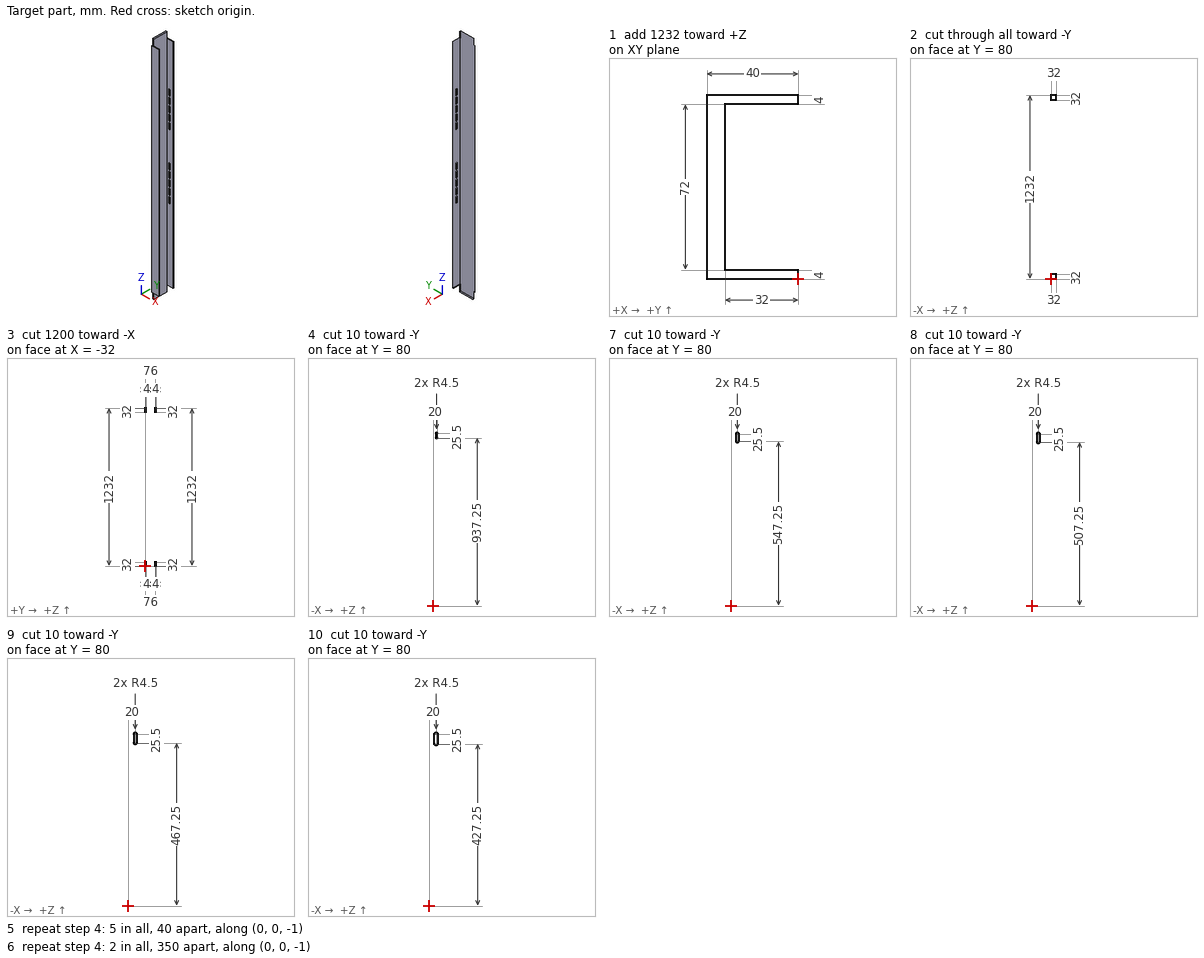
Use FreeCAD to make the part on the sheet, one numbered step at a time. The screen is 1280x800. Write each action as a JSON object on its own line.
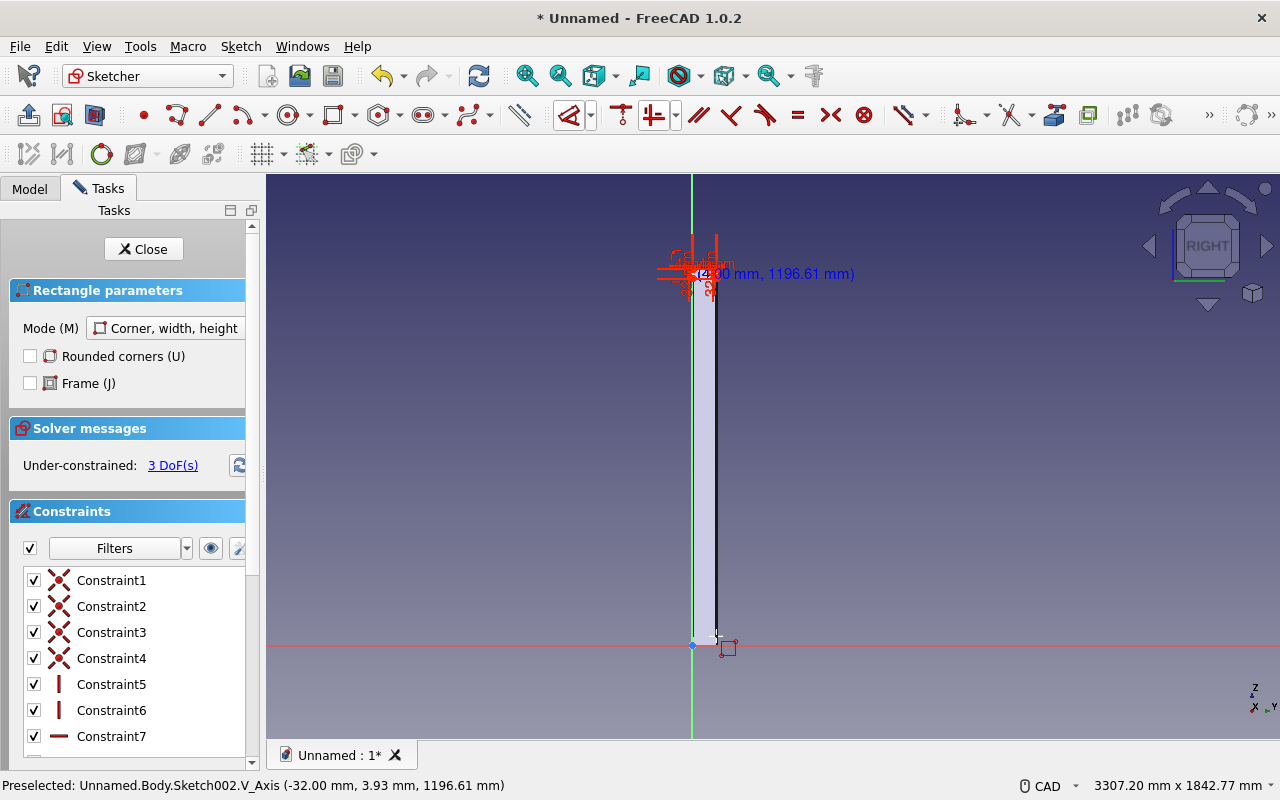
{"action": "scroll", "coordinate": [716, 636], "scroll_direction": "up", "scroll_amount": 3}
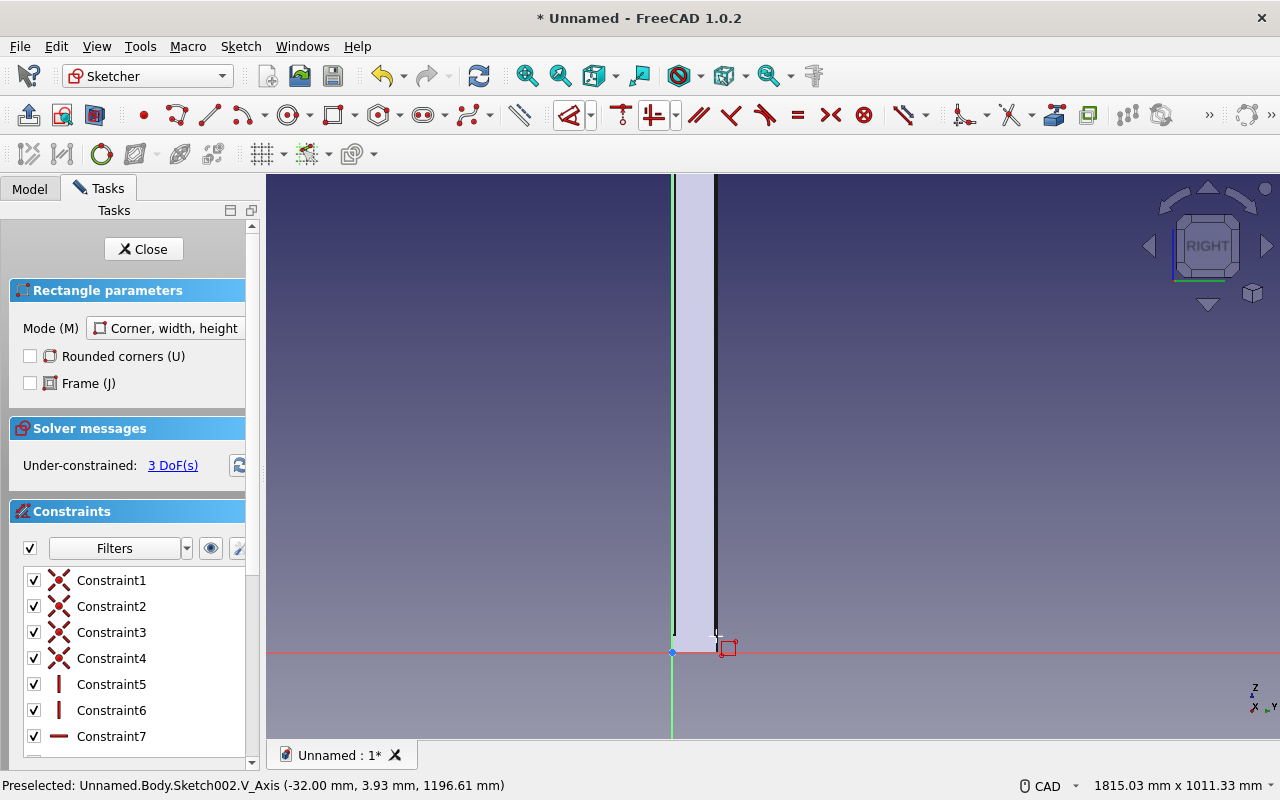
{"action": "left_click", "coordinate": [715, 635]}
{"action": "left_click", "coordinate": [717, 653]}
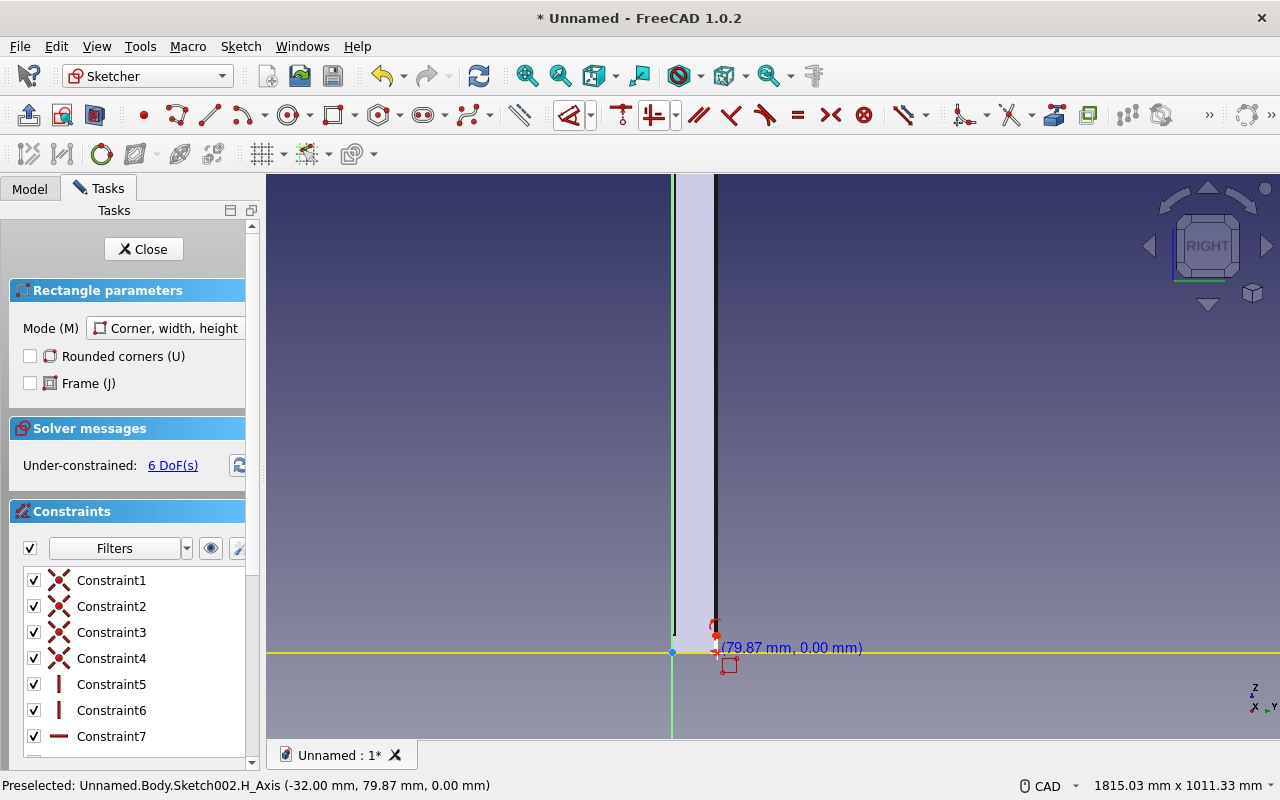
{"action": "scroll", "coordinate": [672, 653], "scroll_direction": "up", "scroll_amount": 10}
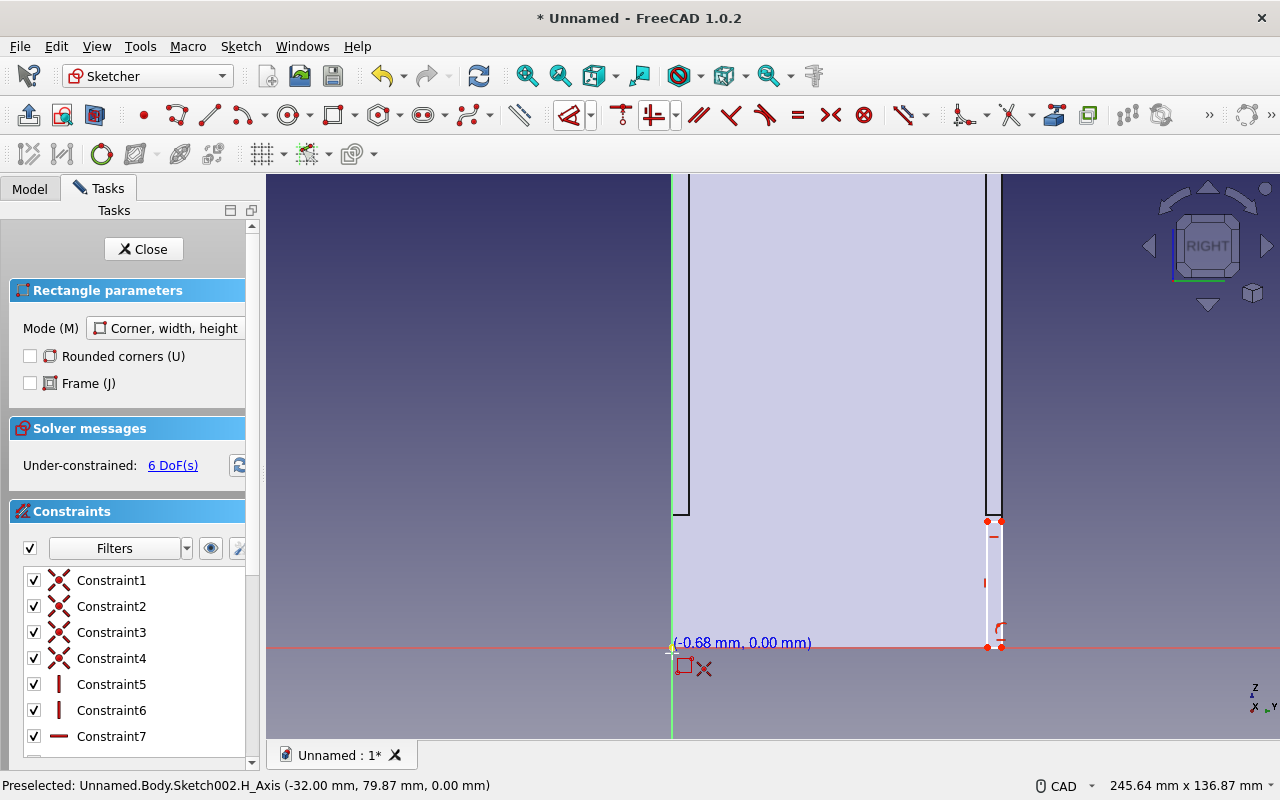
{"action": "scroll", "coordinate": [694, 645], "scroll_direction": "down", "scroll_amount": 13}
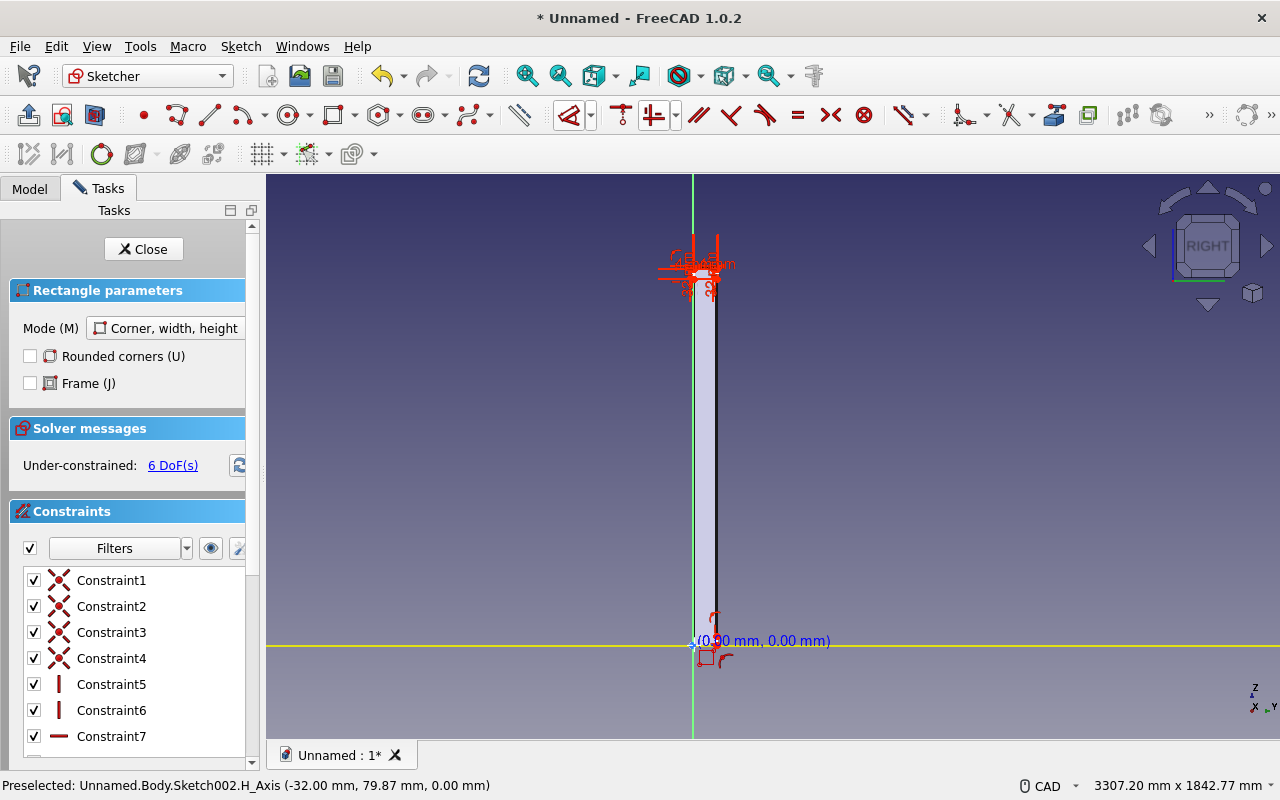
{"action": "left_click", "coordinate": [693, 646]}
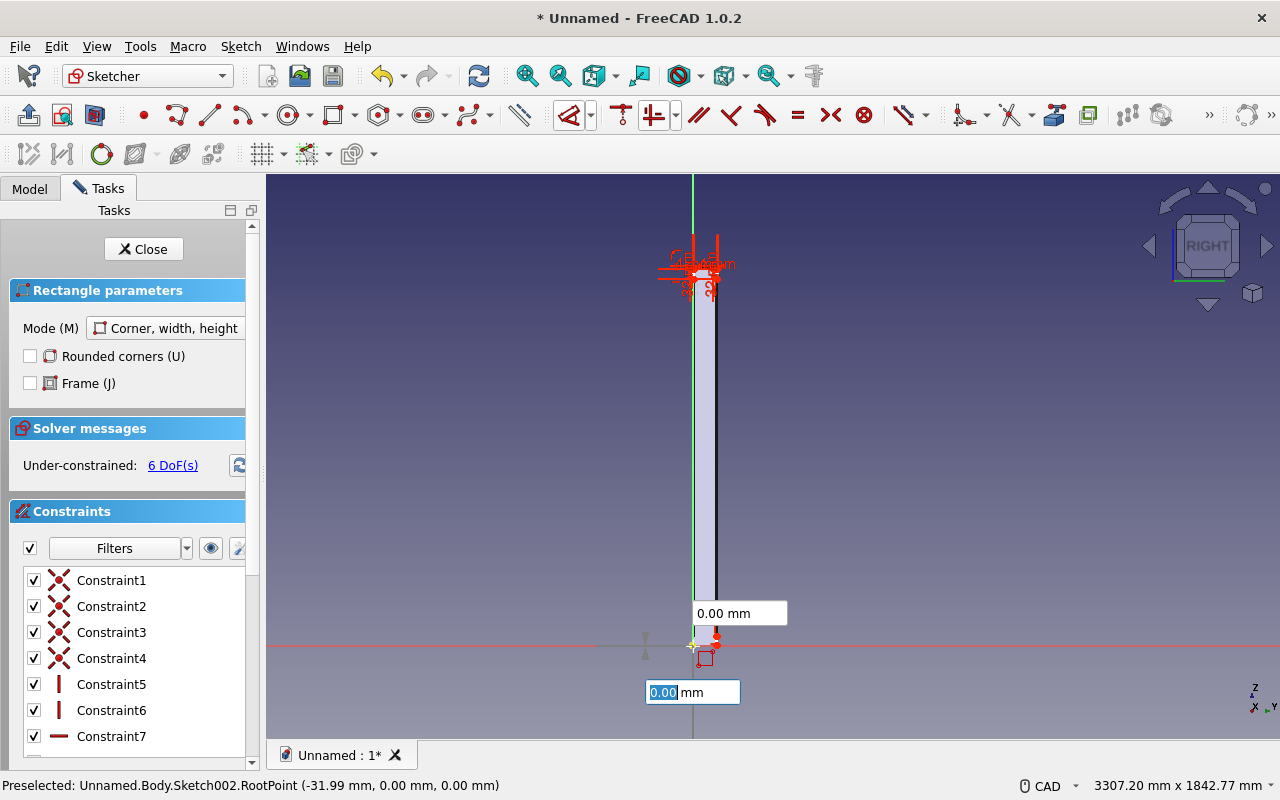
{"action": "scroll", "coordinate": [694, 636], "scroll_direction": "up", "scroll_amount": 13}
{"action": "mouse_move", "coordinate": [689, 628]}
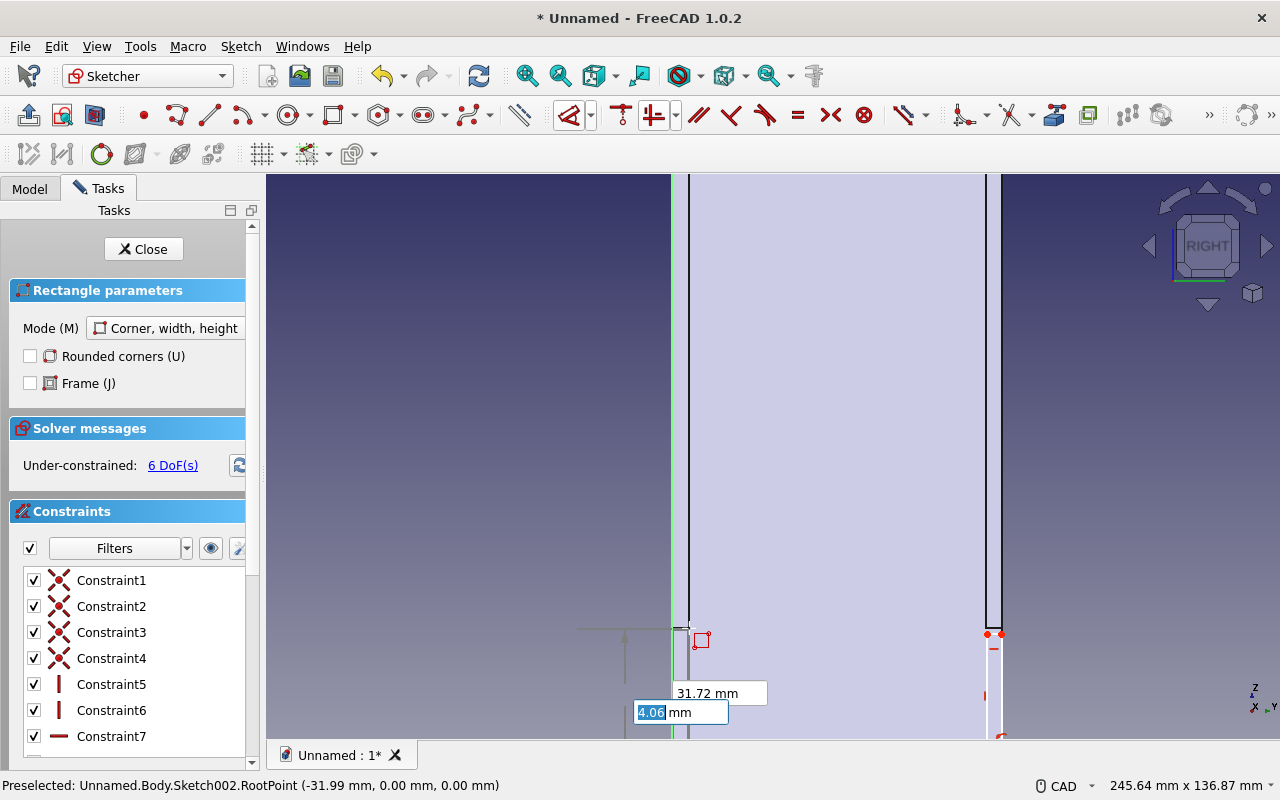
{"action": "type", "text": "4"}
{"action": "key", "text": "Tab"}
{"action": "type", "text": "32"}
{"action": "key", "text": "Return"}
{"action": "key", "text": "Escape"}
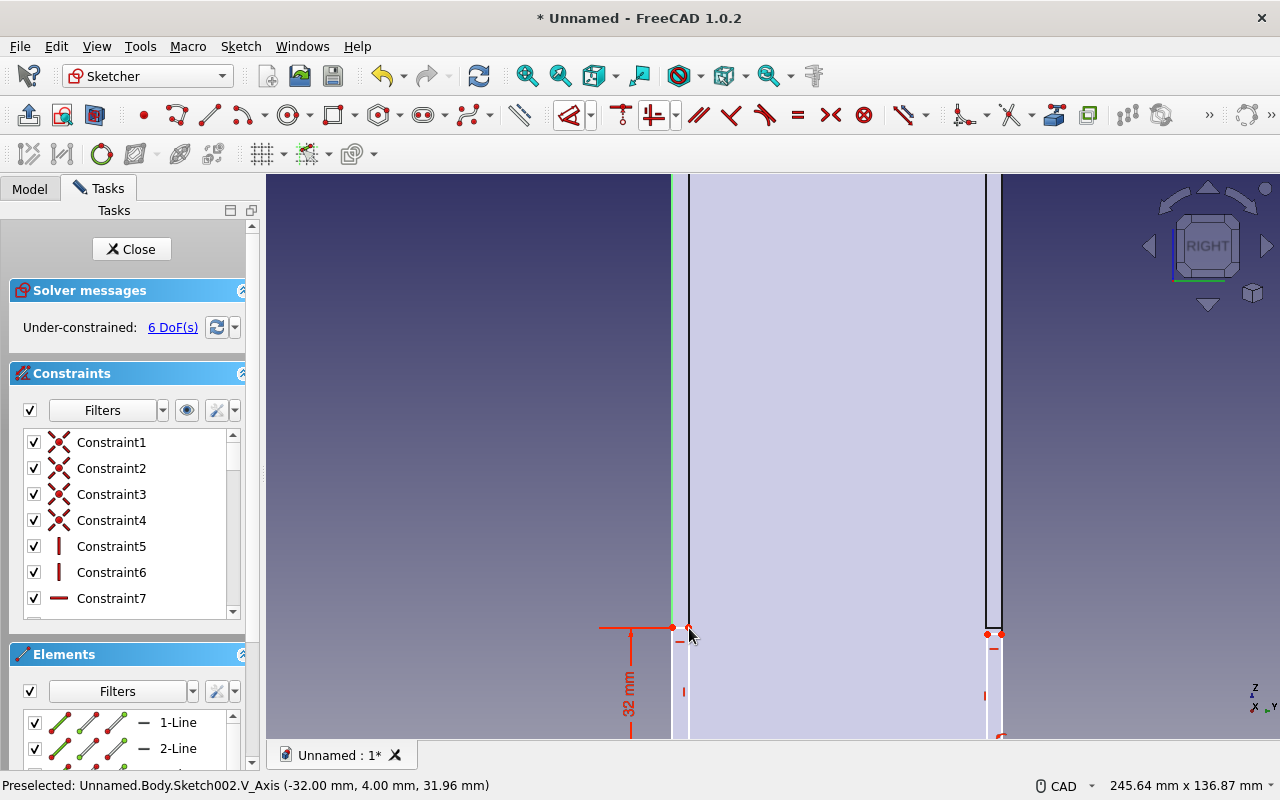
{"action": "scroll", "coordinate": [694, 636], "scroll_direction": "down", "scroll_amount": 13}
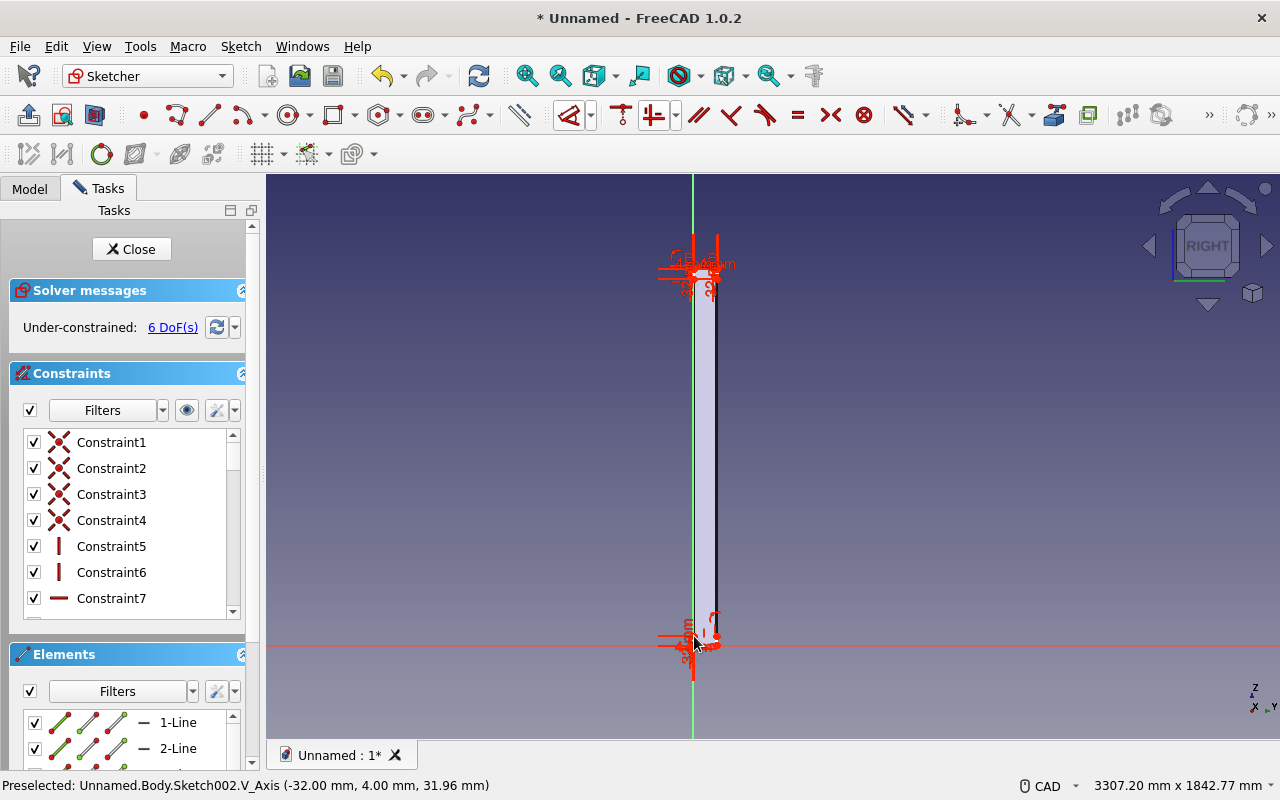
{"action": "scroll", "coordinate": [717, 646], "scroll_direction": "up", "scroll_amount": 18}